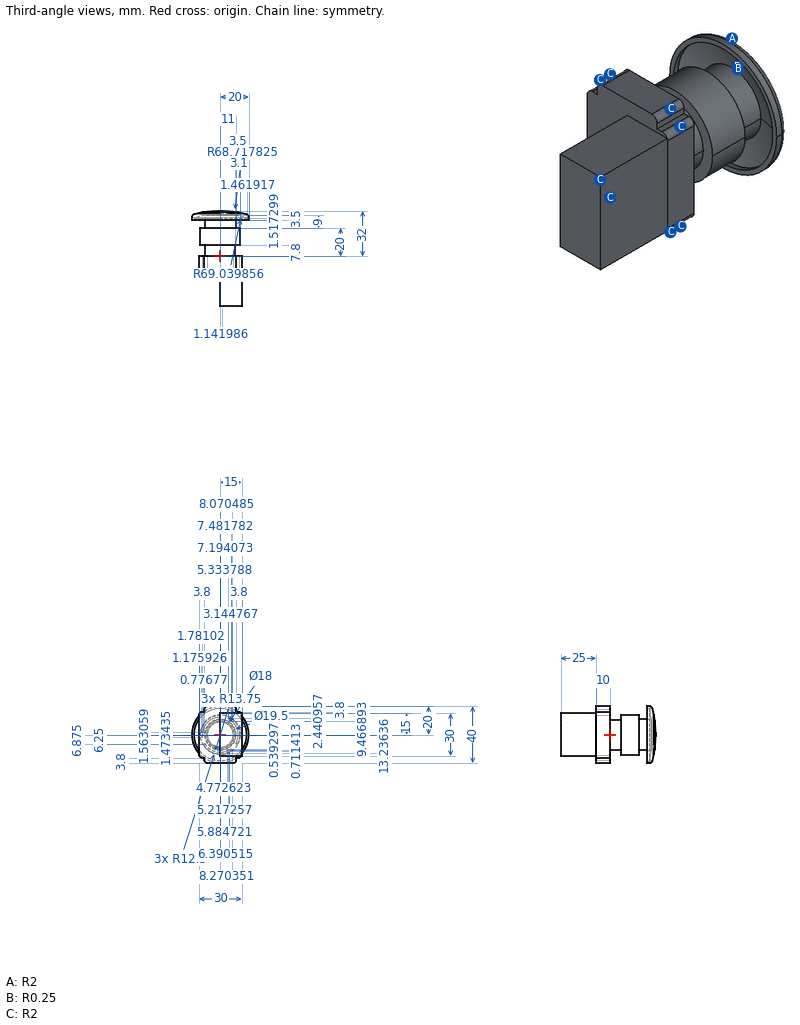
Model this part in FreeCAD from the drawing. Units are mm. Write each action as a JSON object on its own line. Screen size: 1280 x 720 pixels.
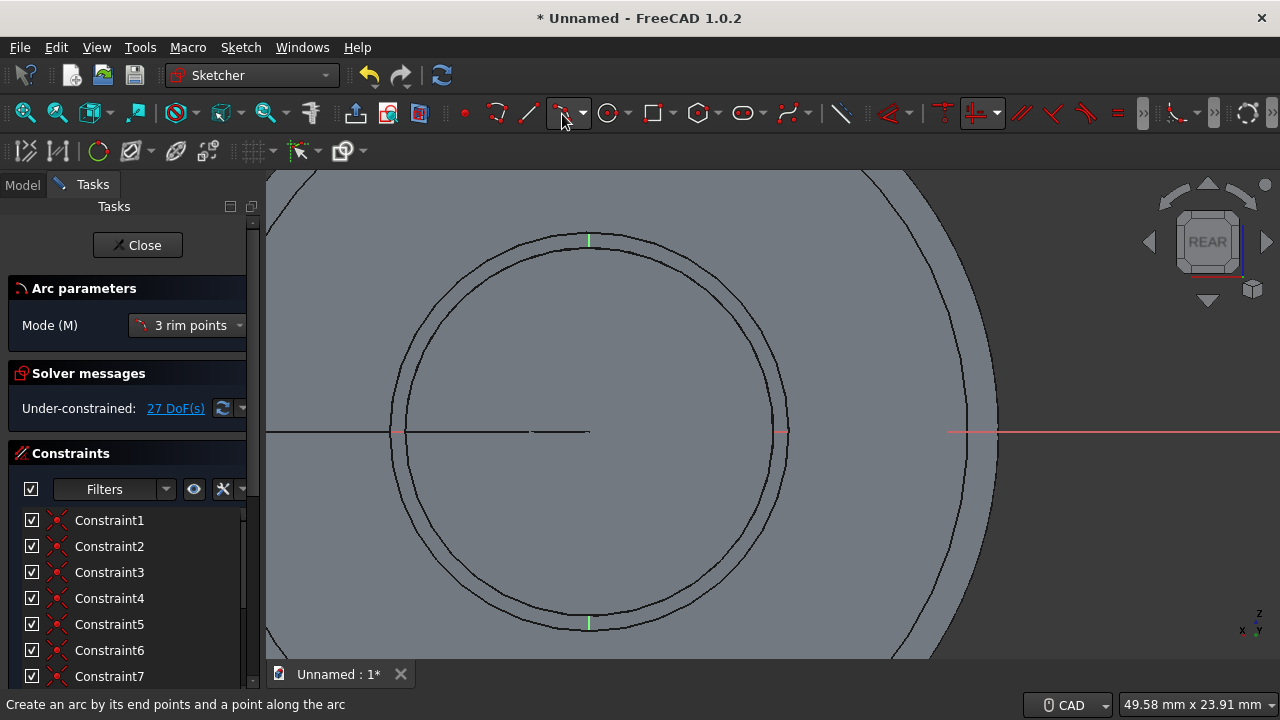
{"action": "scroll", "coordinate": [827, 400], "scroll_direction": "down", "scroll_amount": 3}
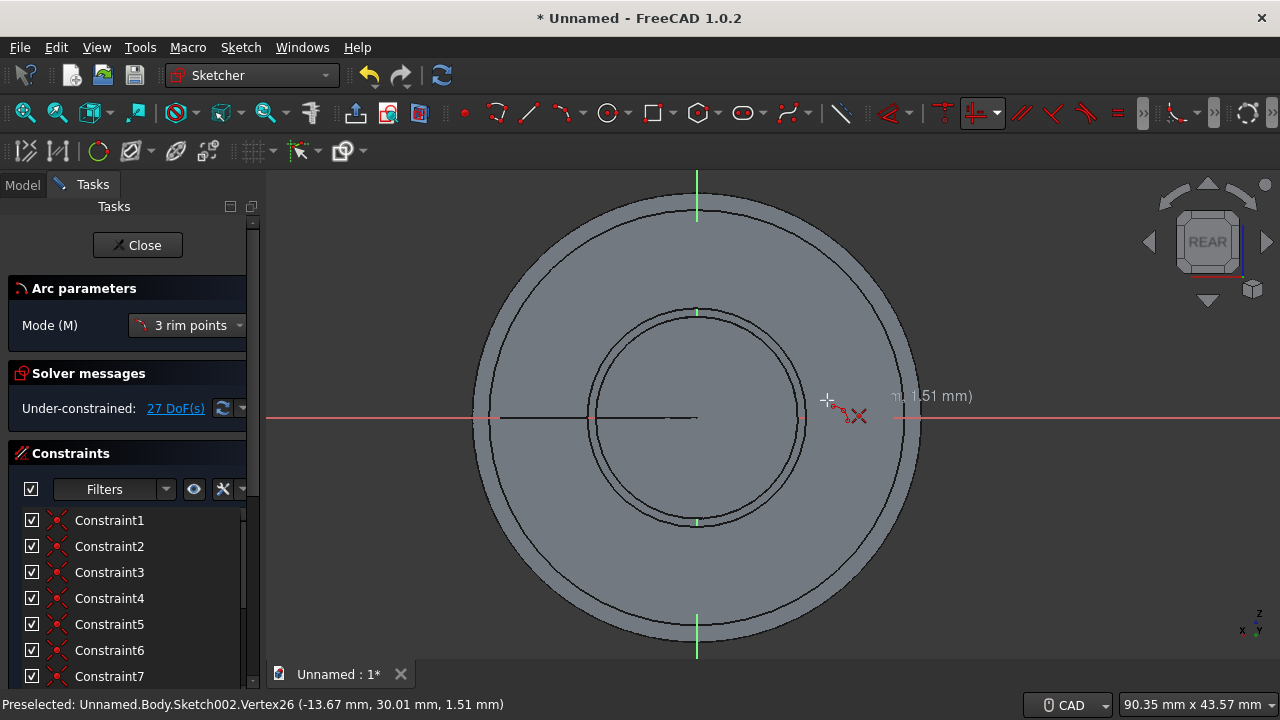
{"action": "scroll", "coordinate": [697, 277], "scroll_direction": "up", "scroll_amount": 5}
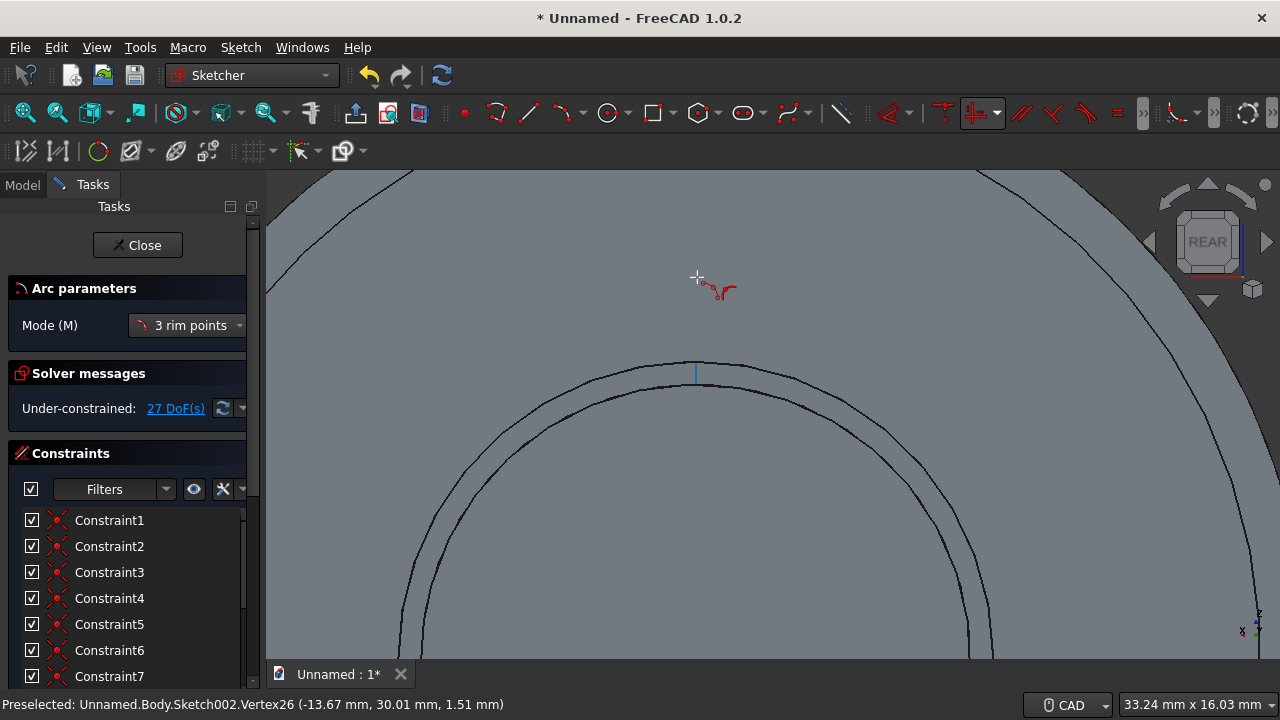
{"action": "left_click", "coordinate": [720, 279]}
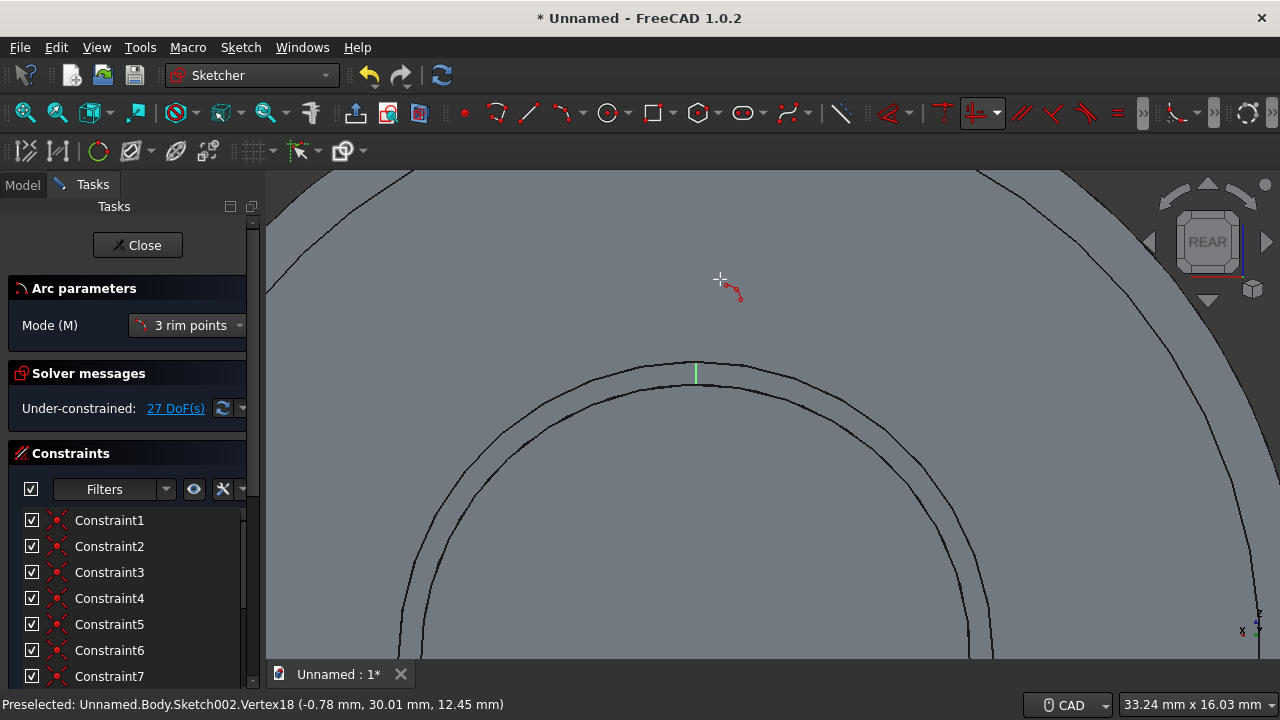
{"action": "scroll", "coordinate": [1074, 611], "scroll_direction": "up", "scroll_amount": 2}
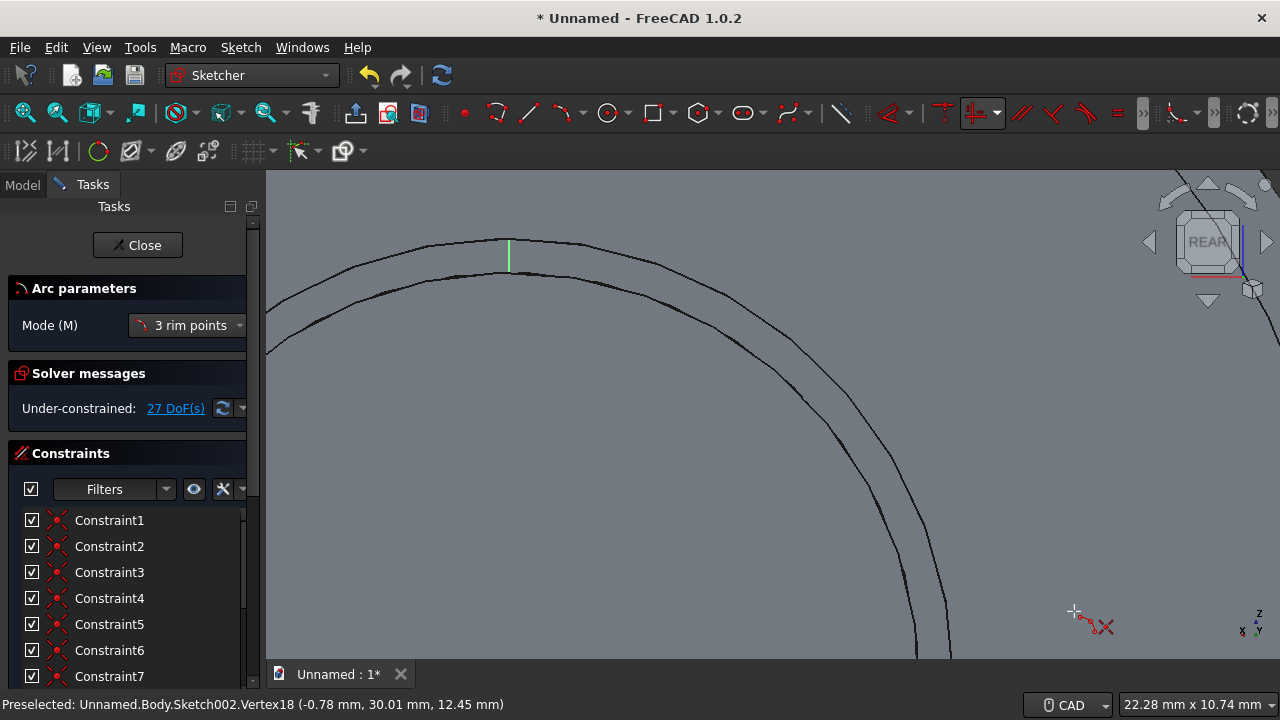
{"action": "left_click", "coordinate": [1072, 615]}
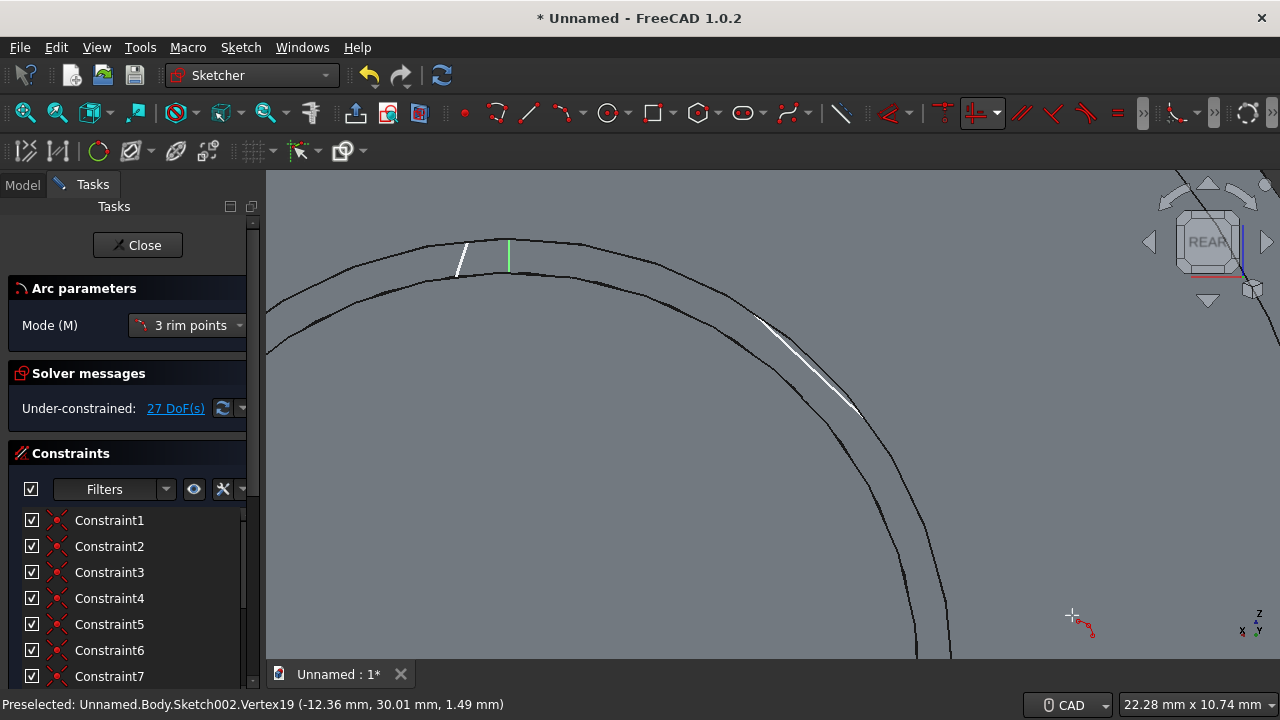
{"action": "scroll", "coordinate": [758, 331], "scroll_direction": "down", "scroll_amount": 7}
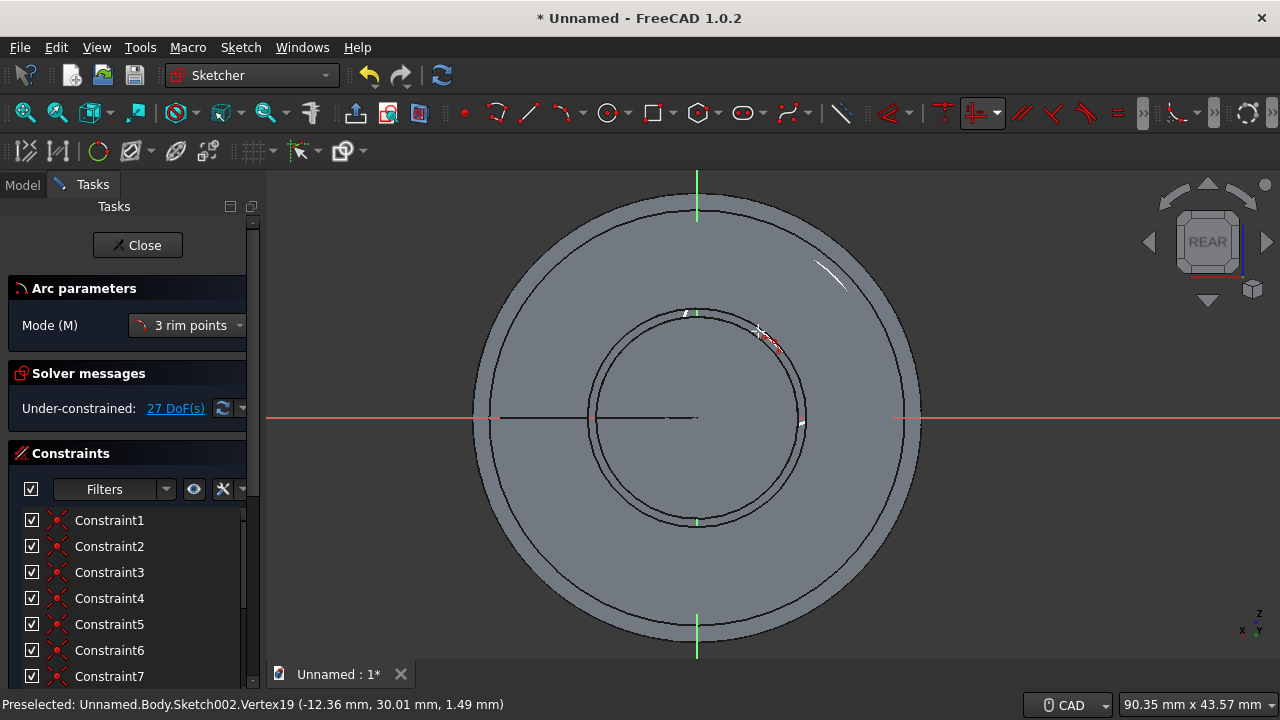
{"action": "left_click", "coordinate": [790, 313]}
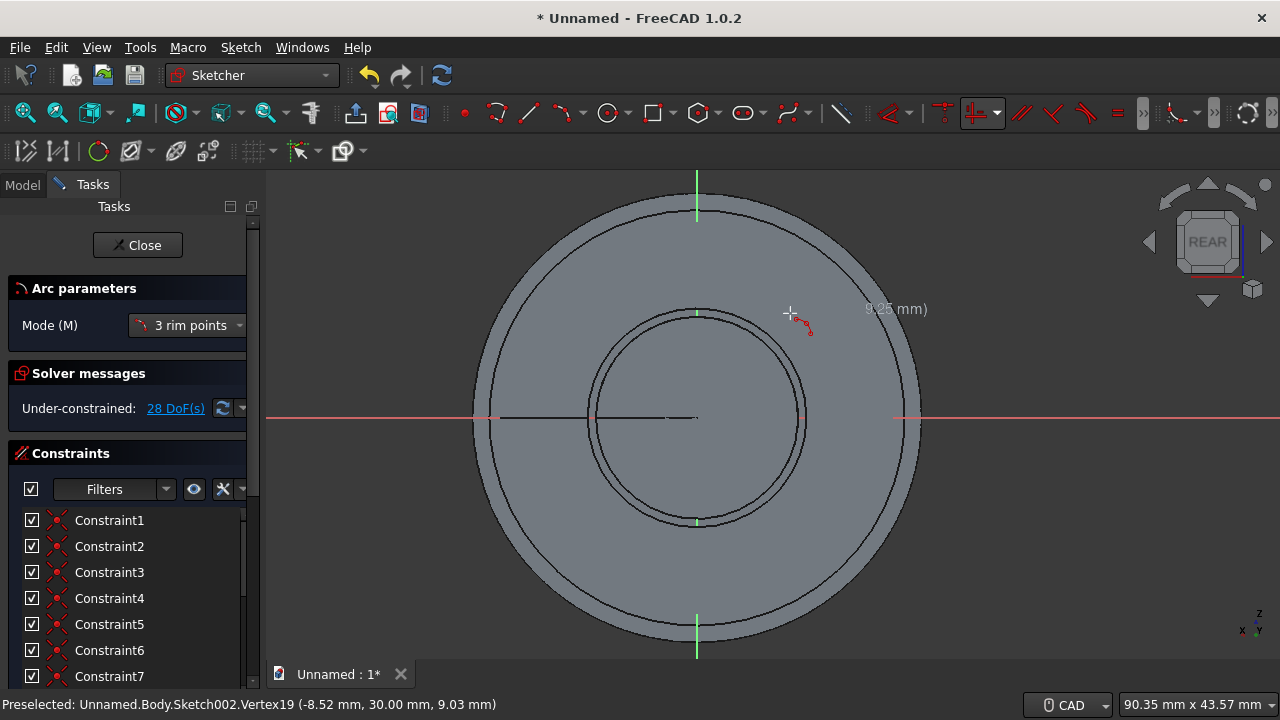
{"action": "scroll", "coordinate": [850, 400], "scroll_direction": "up", "scroll_amount": 5}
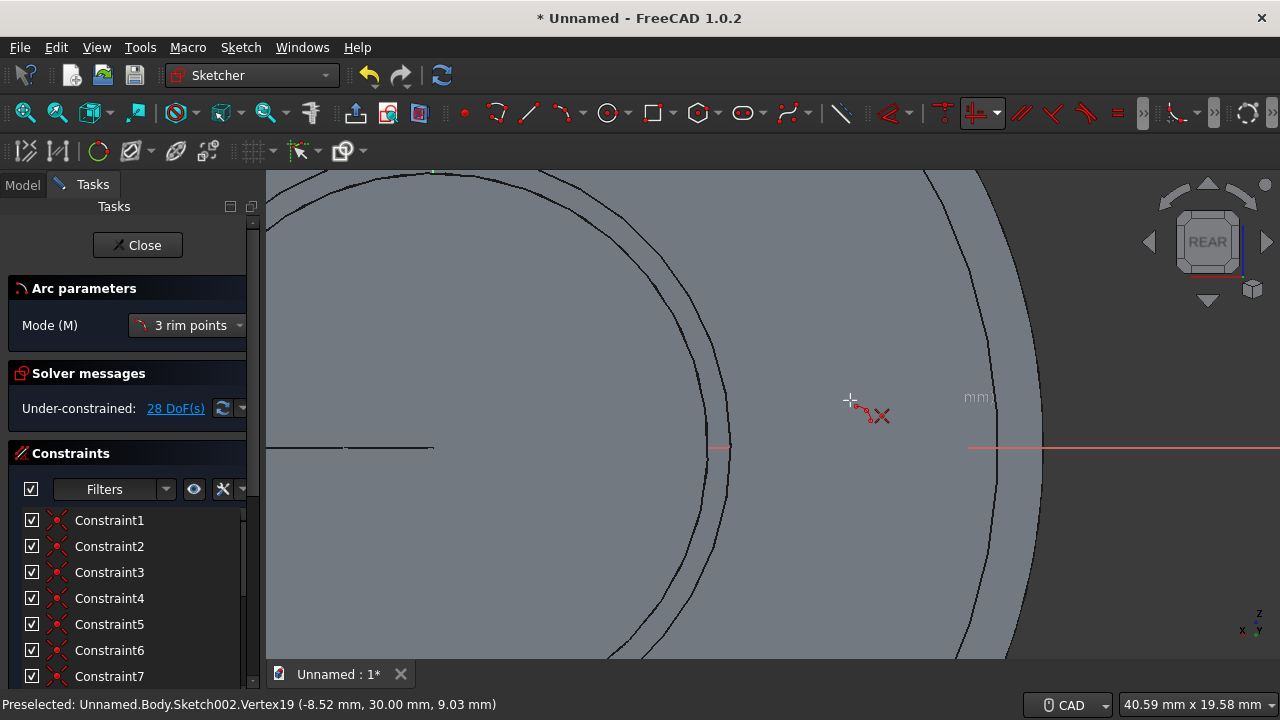
{"action": "left_click", "coordinate": [850, 402]}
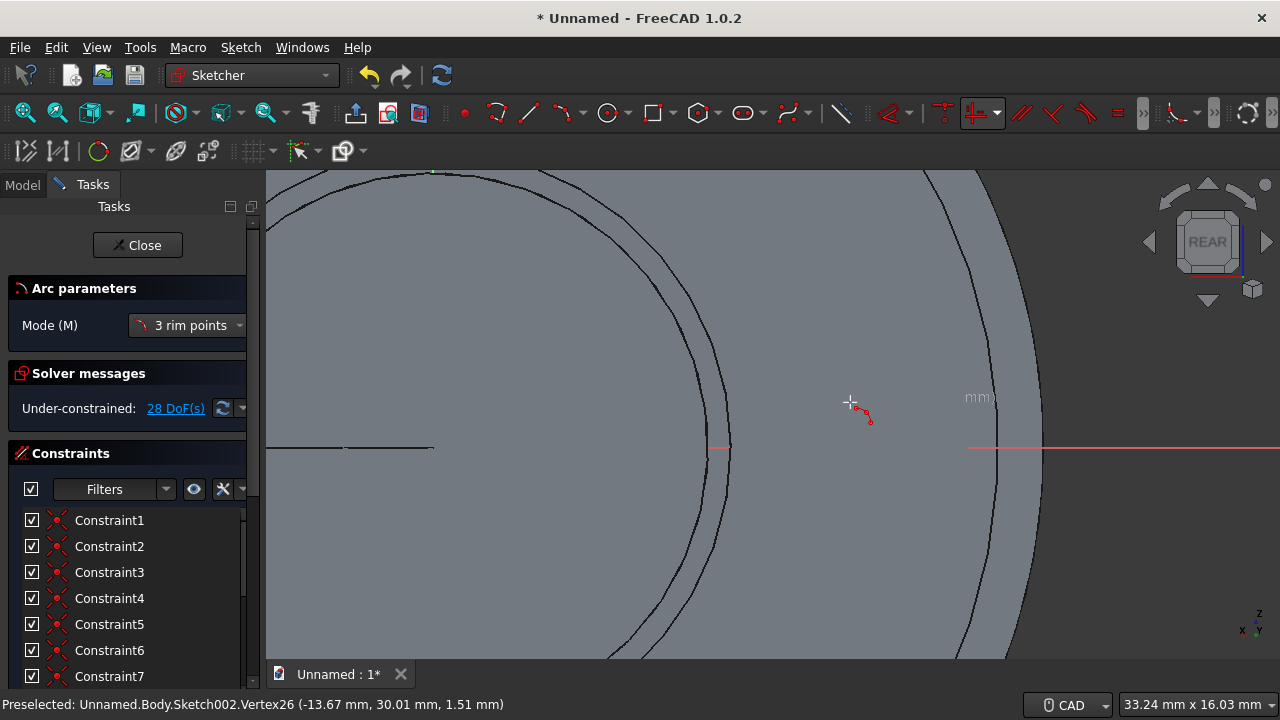
{"action": "scroll", "coordinate": [850, 400], "scroll_direction": "down", "scroll_amount": 5}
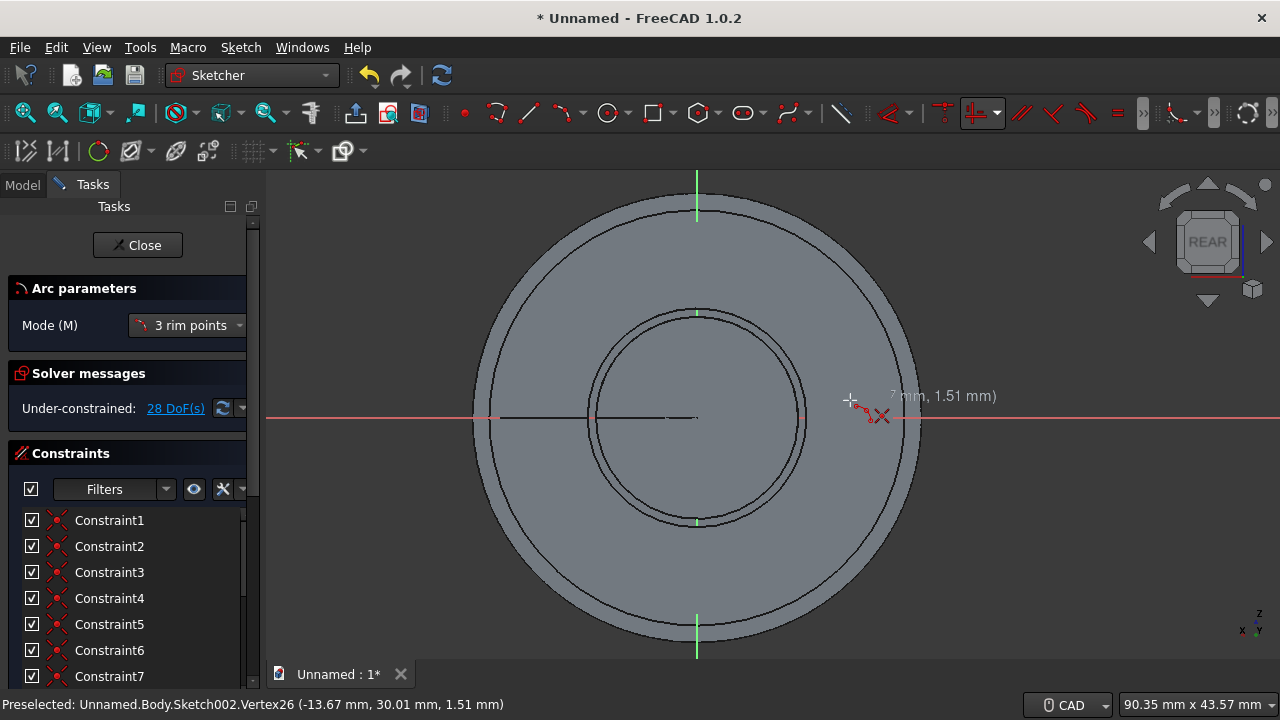
{"action": "scroll", "coordinate": [697, 264], "scroll_direction": "up", "scroll_amount": 5}